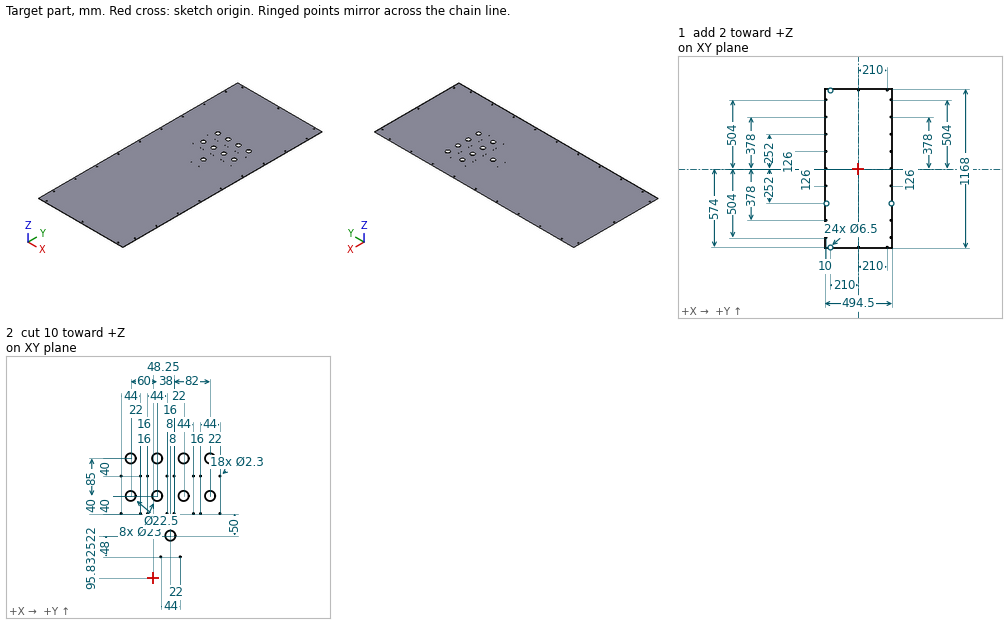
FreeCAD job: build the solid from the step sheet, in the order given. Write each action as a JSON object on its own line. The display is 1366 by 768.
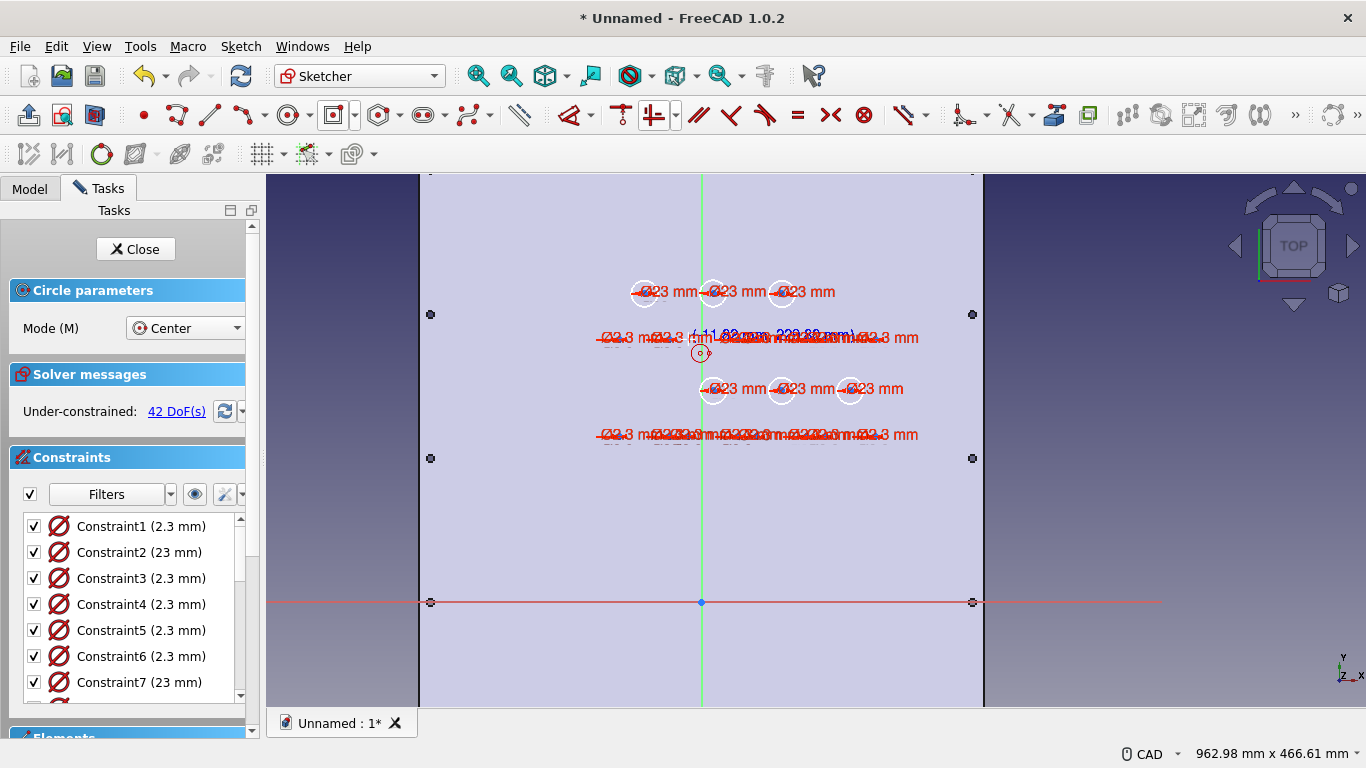
{"action": "left_click", "coordinate": [688, 339]}
{"action": "mouse_move", "coordinate": [687, 338]}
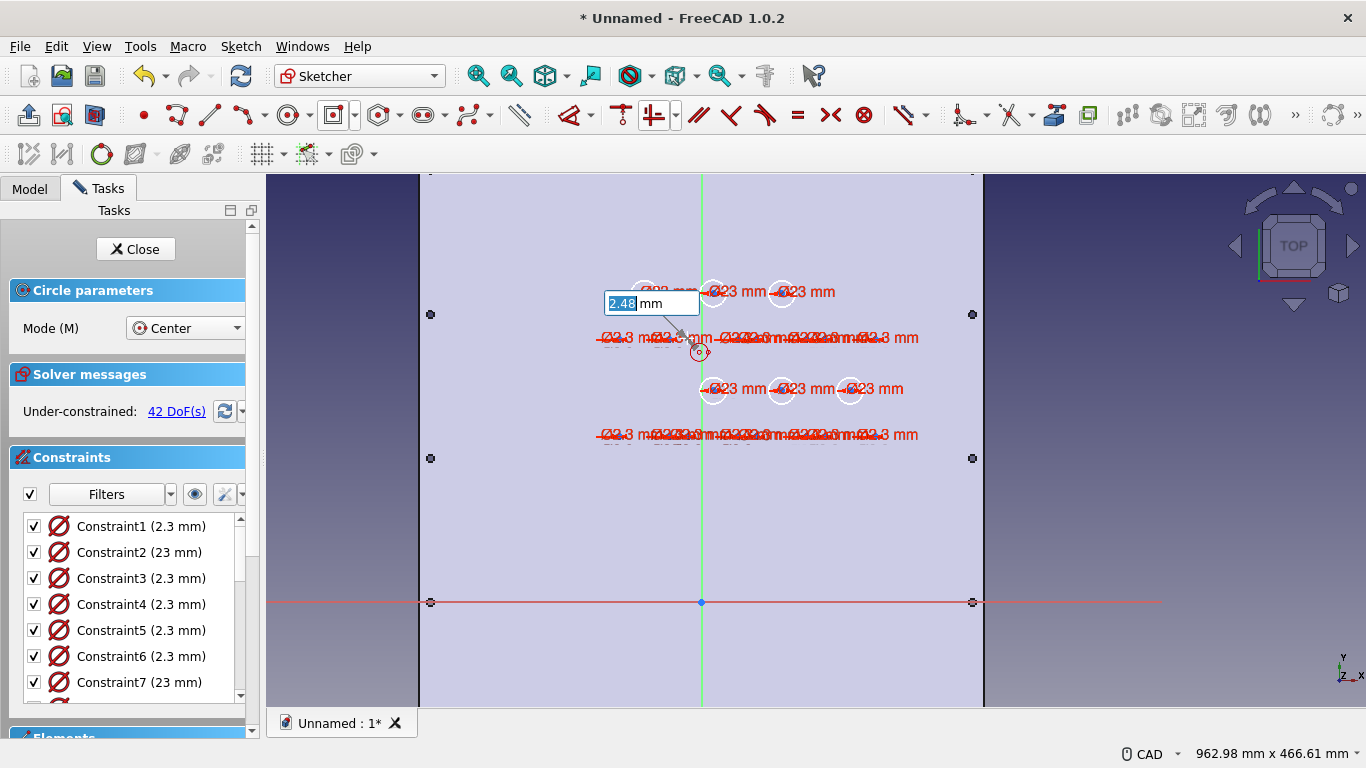
{"action": "type", "text": "2.3"}
{"action": "key", "text": "Return"}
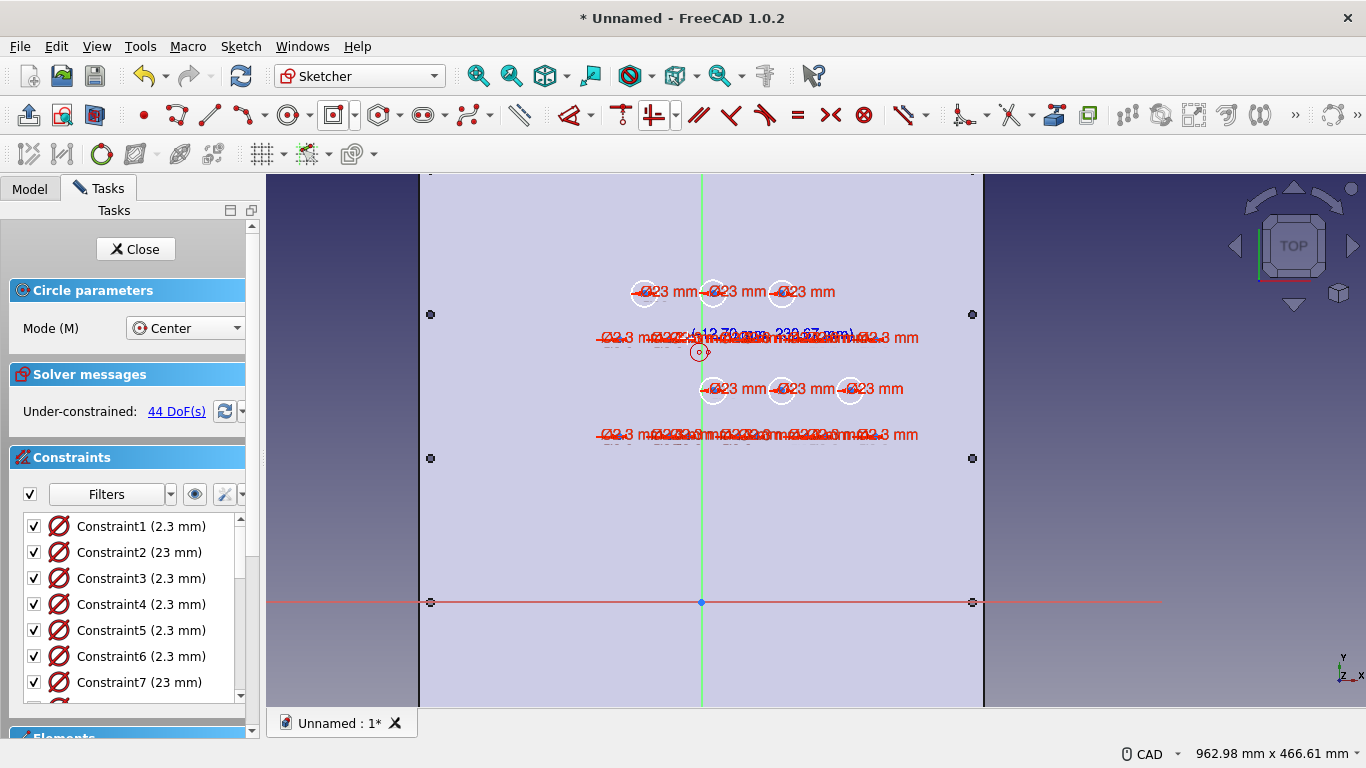
{"action": "scroll", "coordinate": [747, 493], "scroll_direction": "up", "scroll_amount": 3}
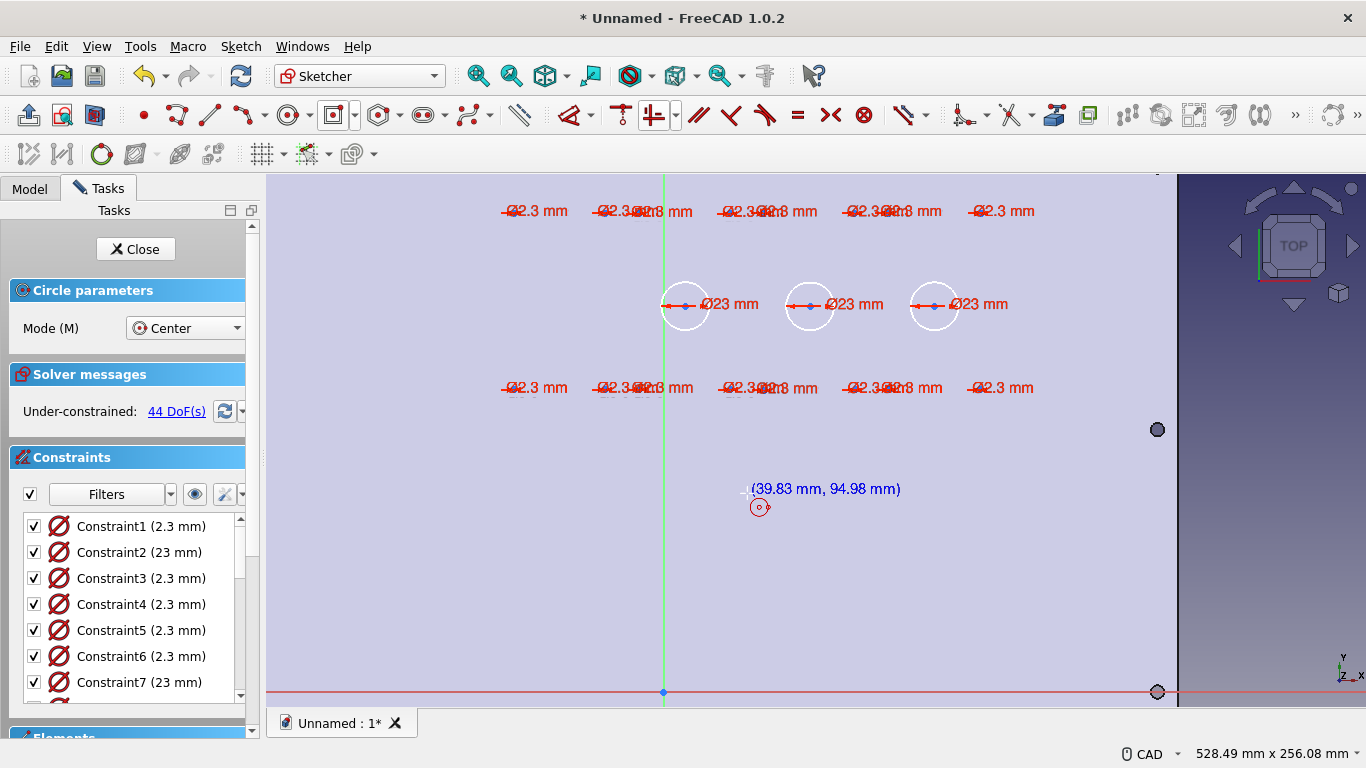
{"action": "left_click", "coordinate": [748, 493]}
{"action": "mouse_move", "coordinate": [764, 476]}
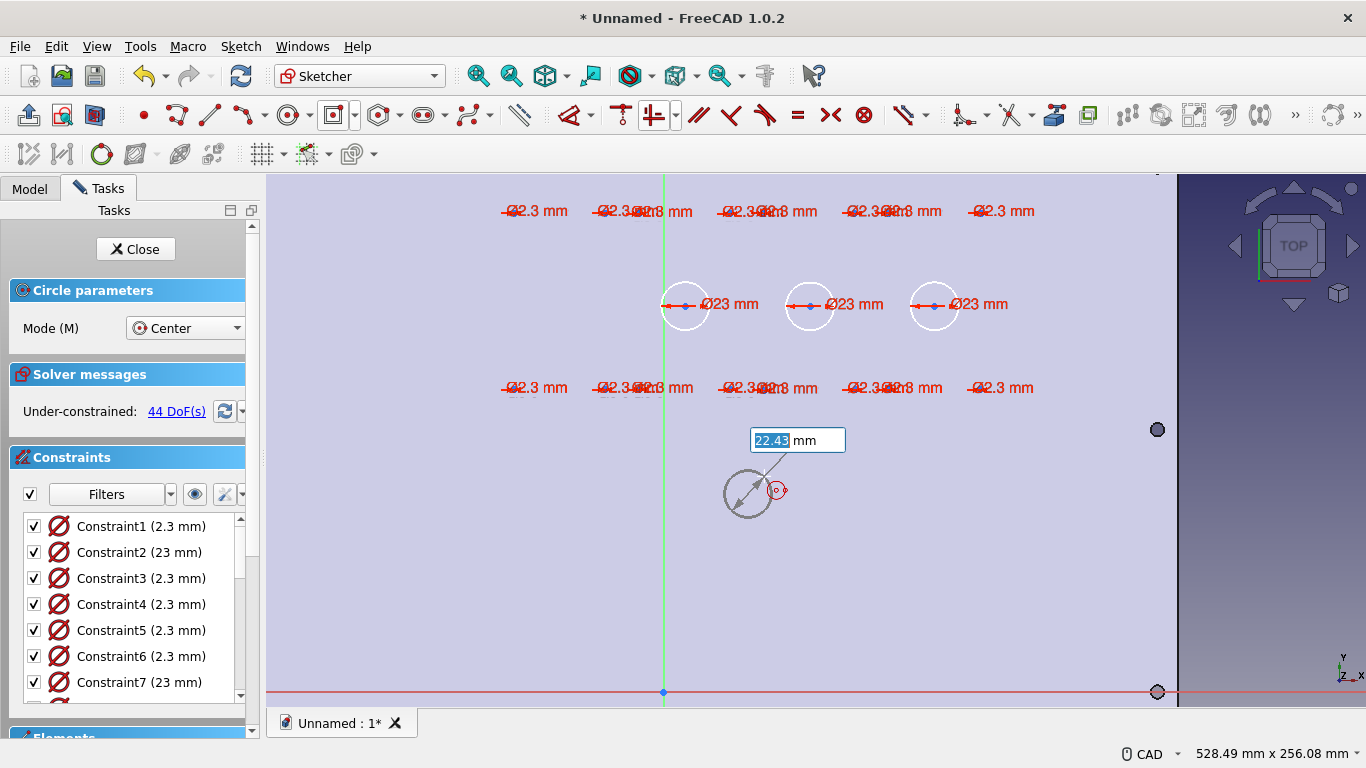
{"action": "type", "text": "23"}
{"action": "key", "text": "Return"}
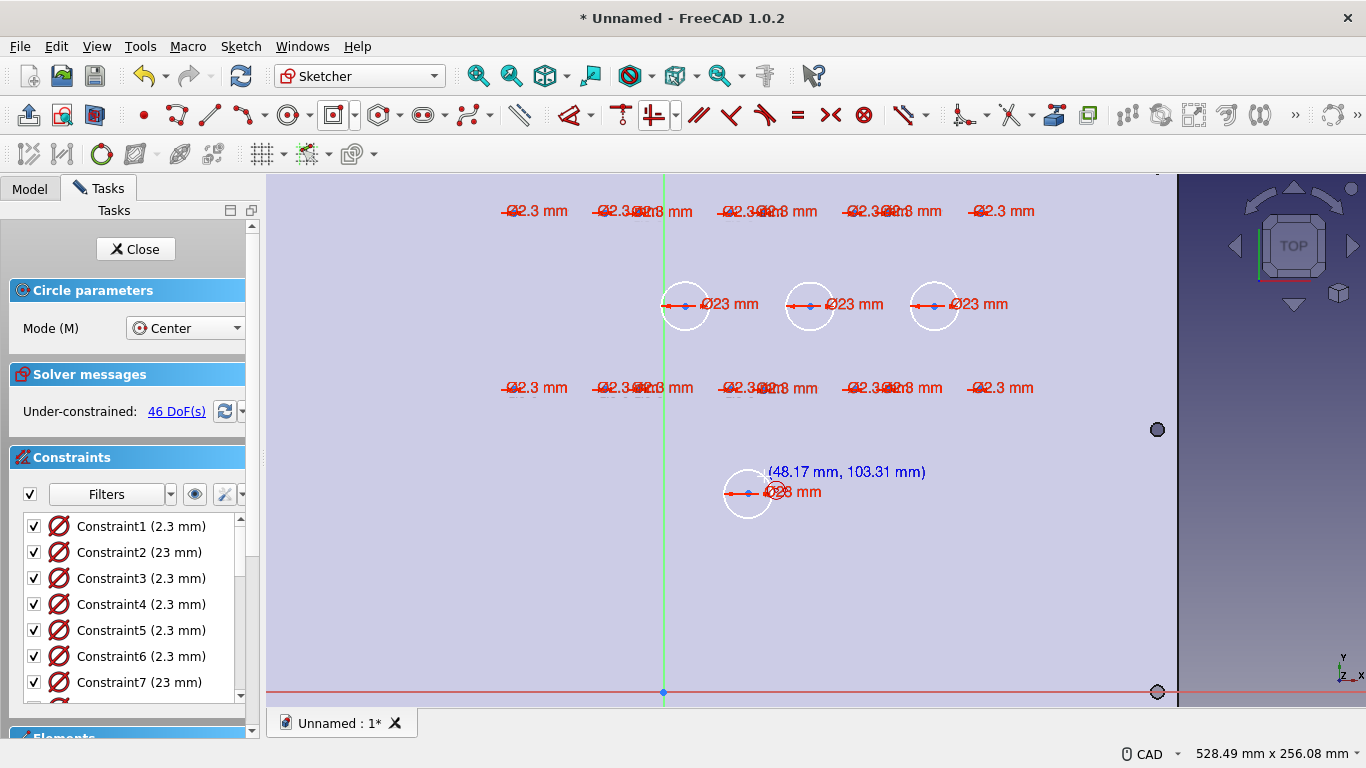
{"action": "scroll", "coordinate": [793, 592], "scroll_direction": "up", "scroll_amount": 12}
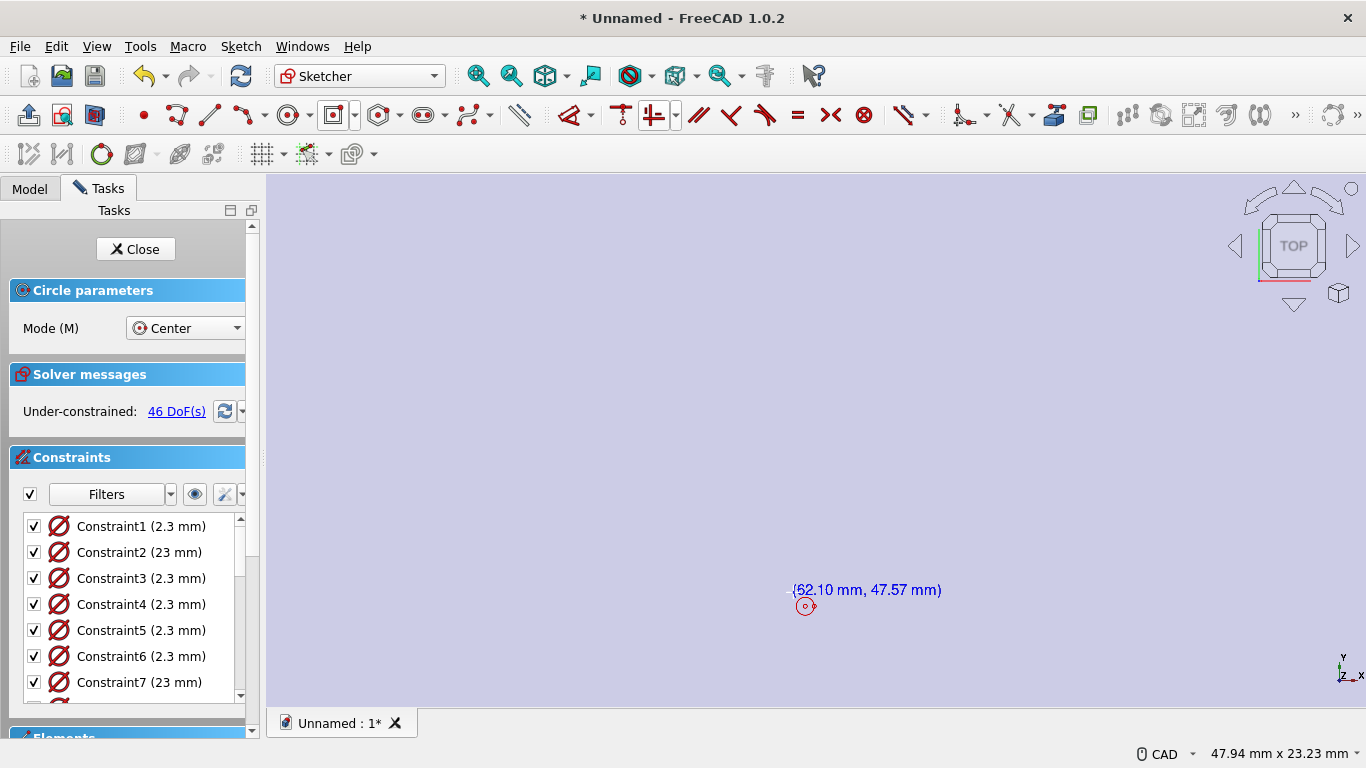
{"action": "scroll", "coordinate": [772, 545], "scroll_direction": "down", "scroll_amount": 15}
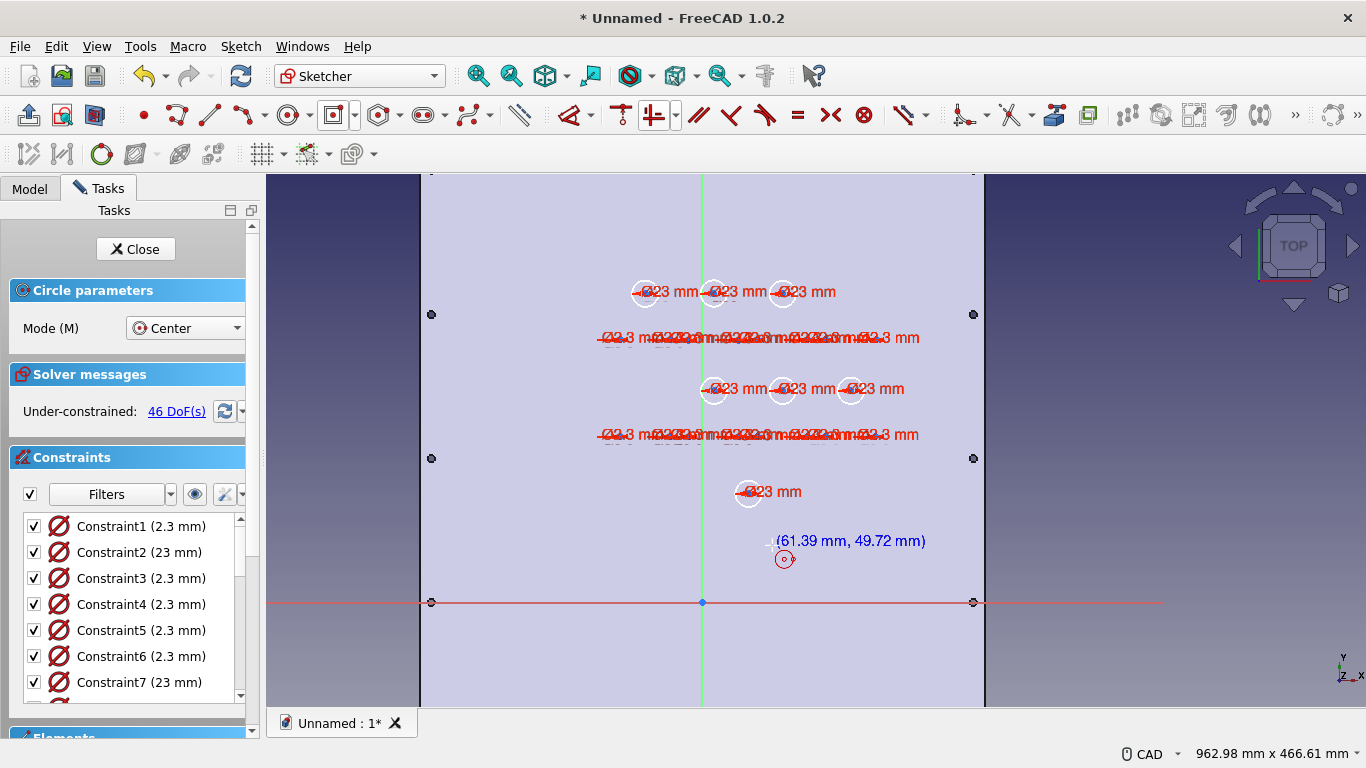
{"action": "left_click", "coordinate": [773, 548]}
{"action": "mouse_move", "coordinate": [774, 547]}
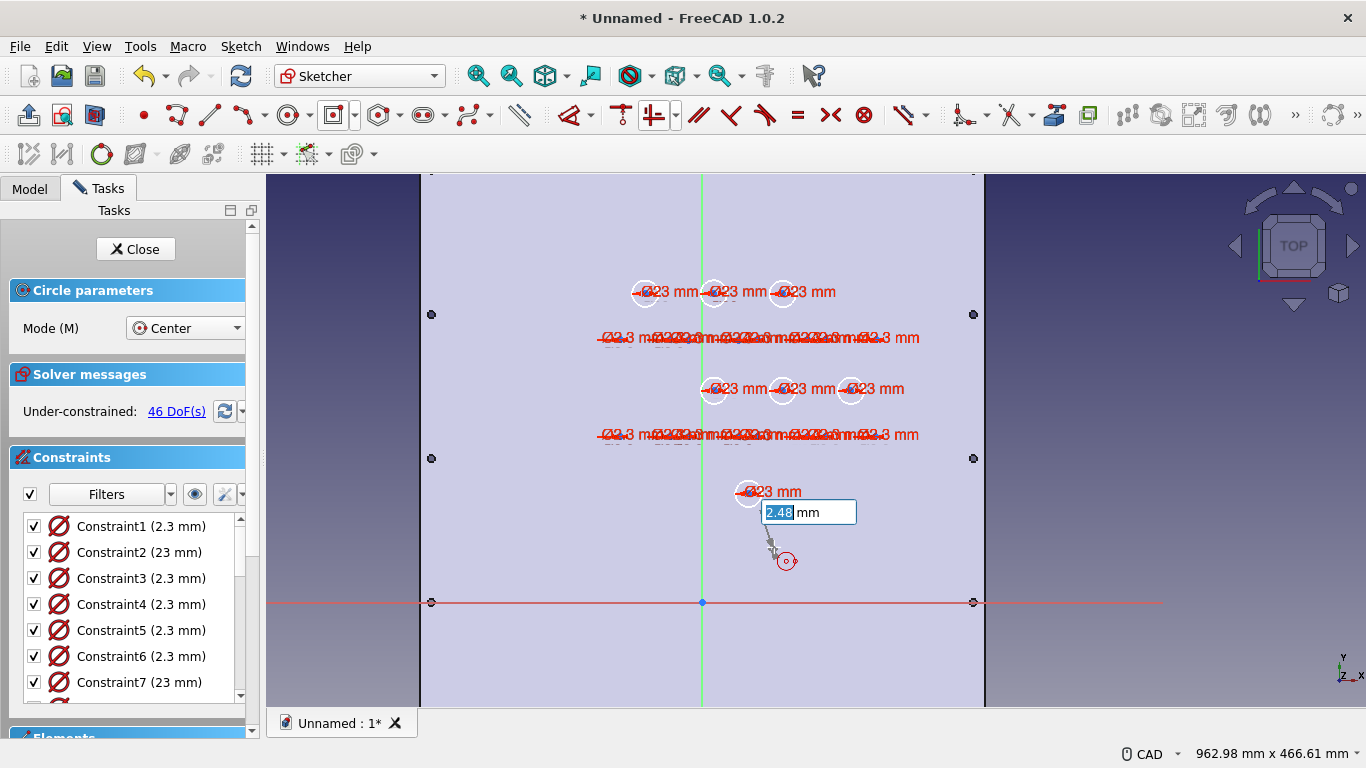
{"action": "type", "text": "2.3"}
{"action": "key", "text": "Return"}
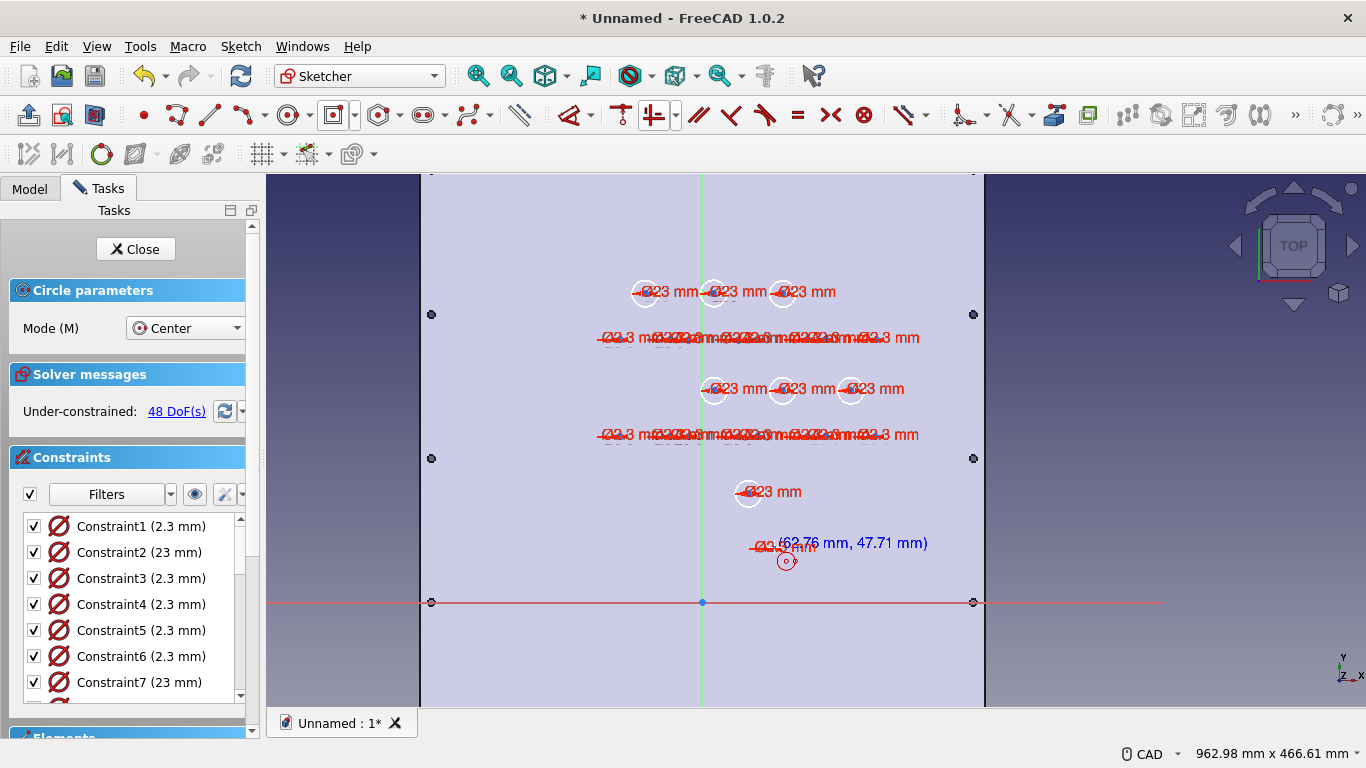
{"action": "scroll", "coordinate": [723, 548], "scroll_direction": "up", "scroll_amount": 15}